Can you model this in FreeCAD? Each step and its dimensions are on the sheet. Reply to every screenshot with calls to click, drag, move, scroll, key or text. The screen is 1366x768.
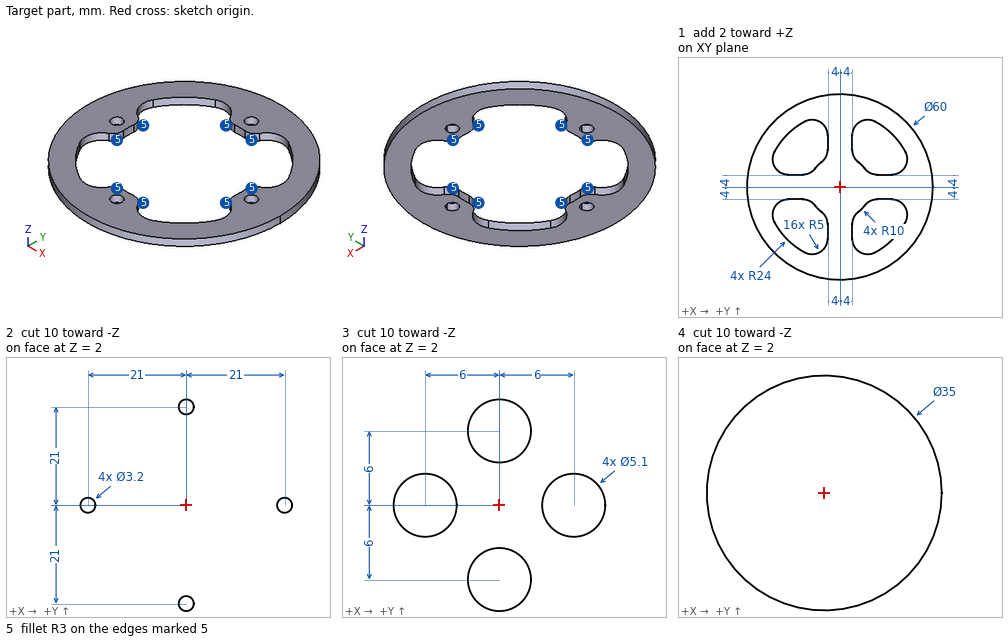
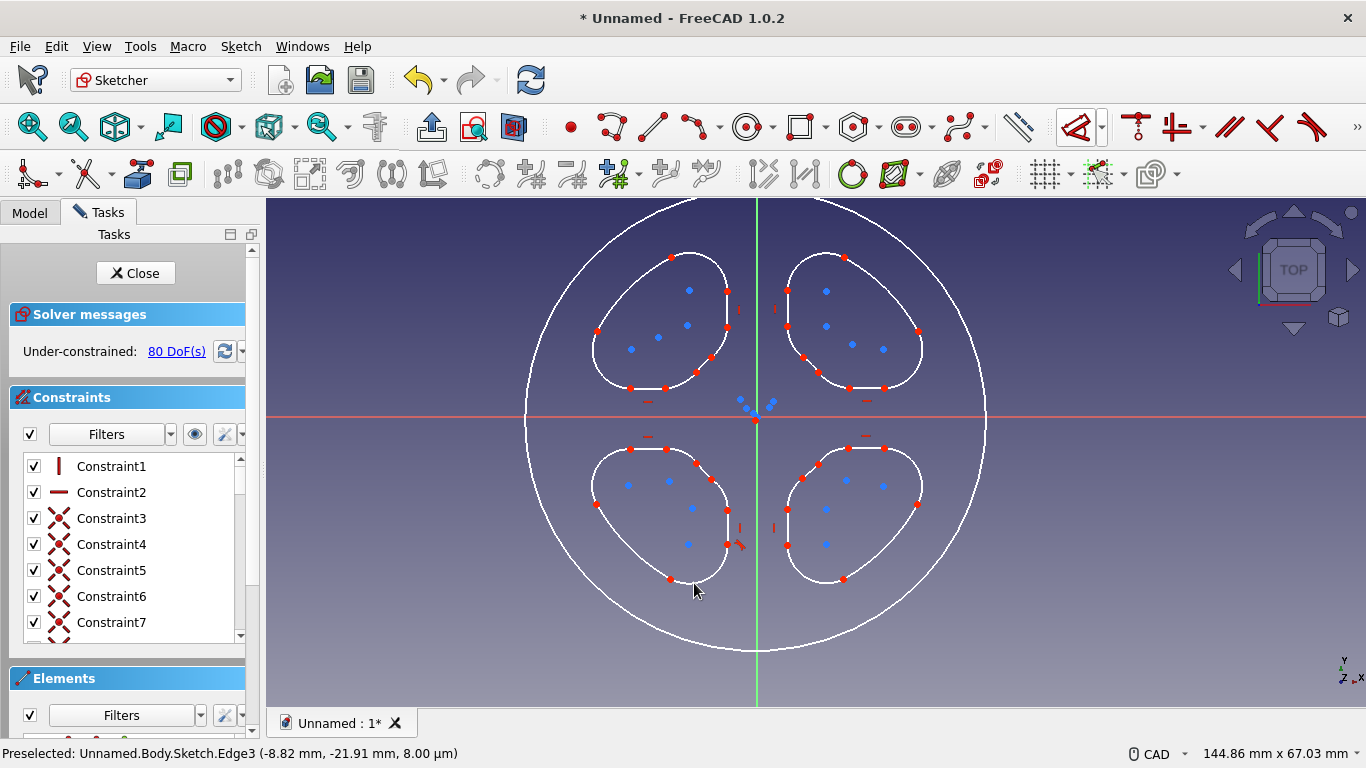
scroll(728, 521, up, 2)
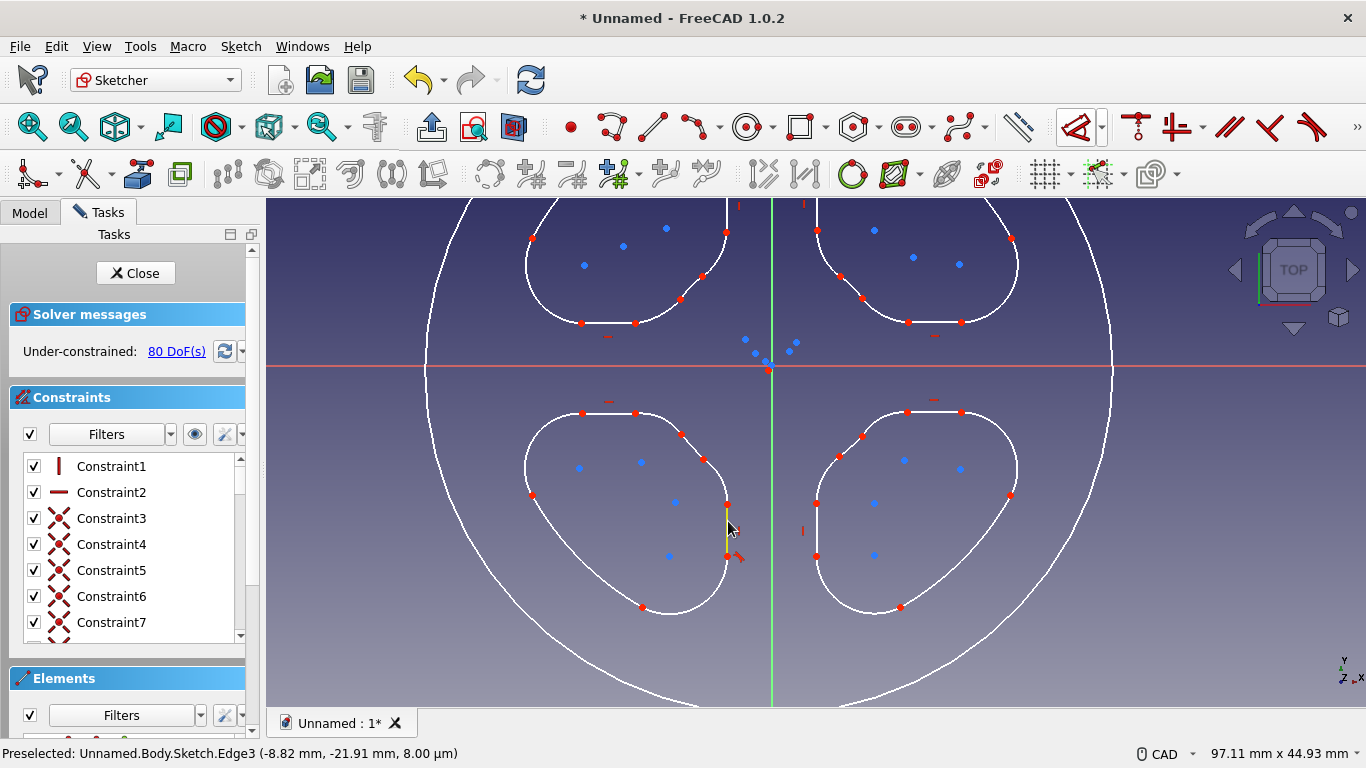
click(727, 520)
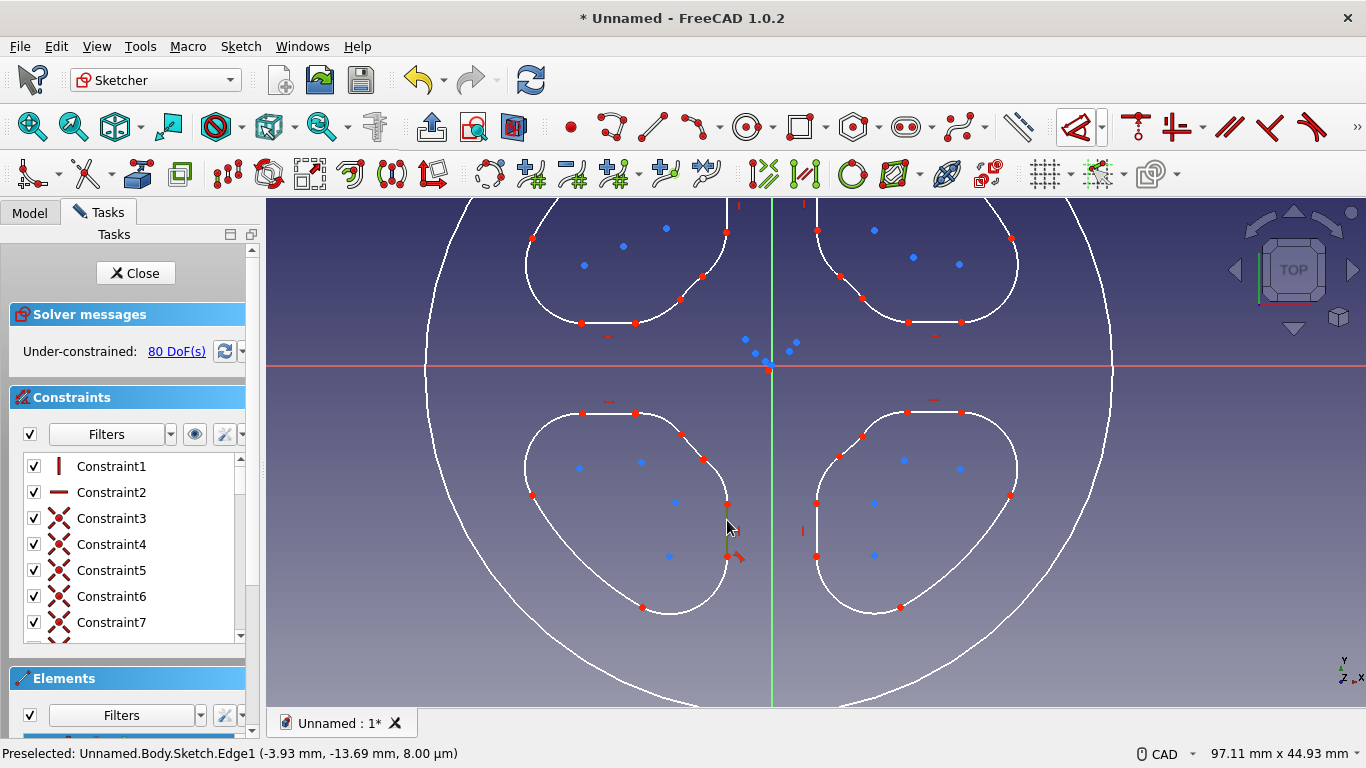
click(725, 489)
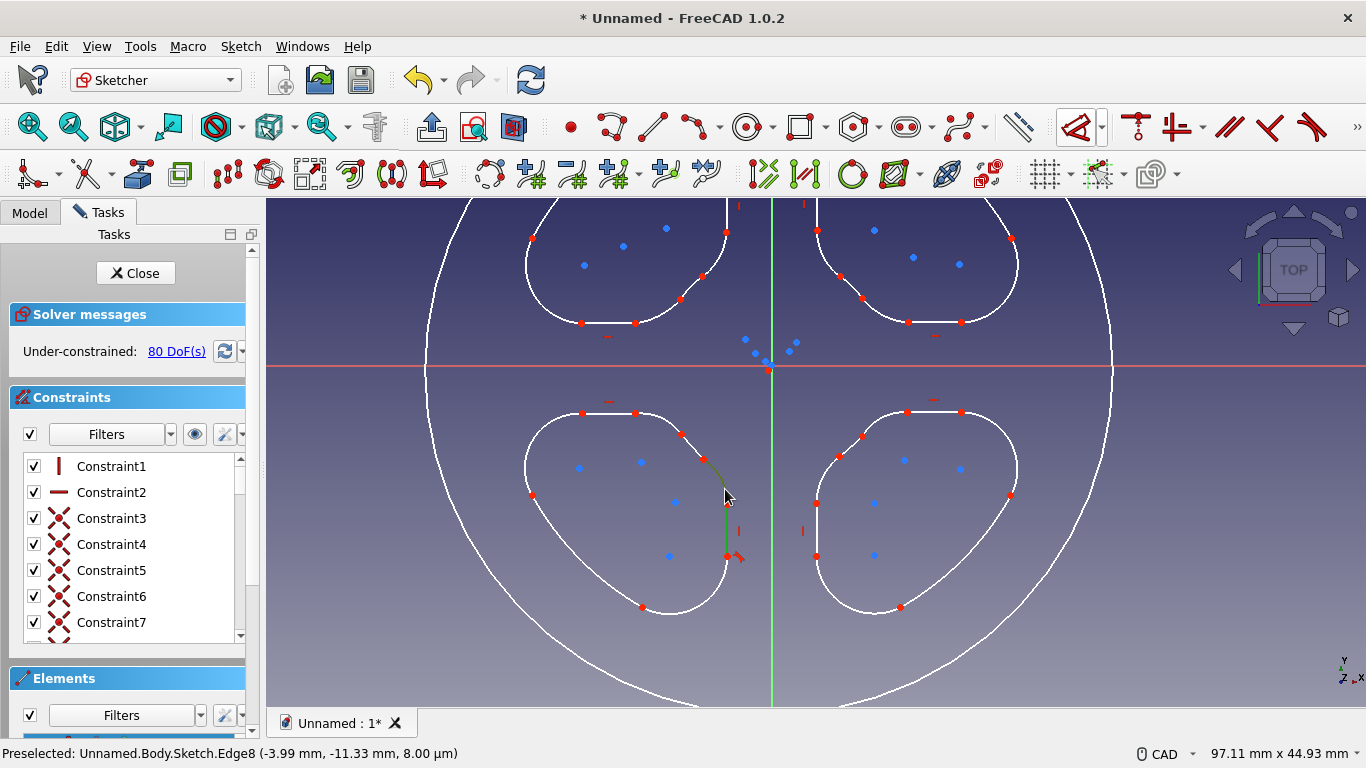
click(1312, 128)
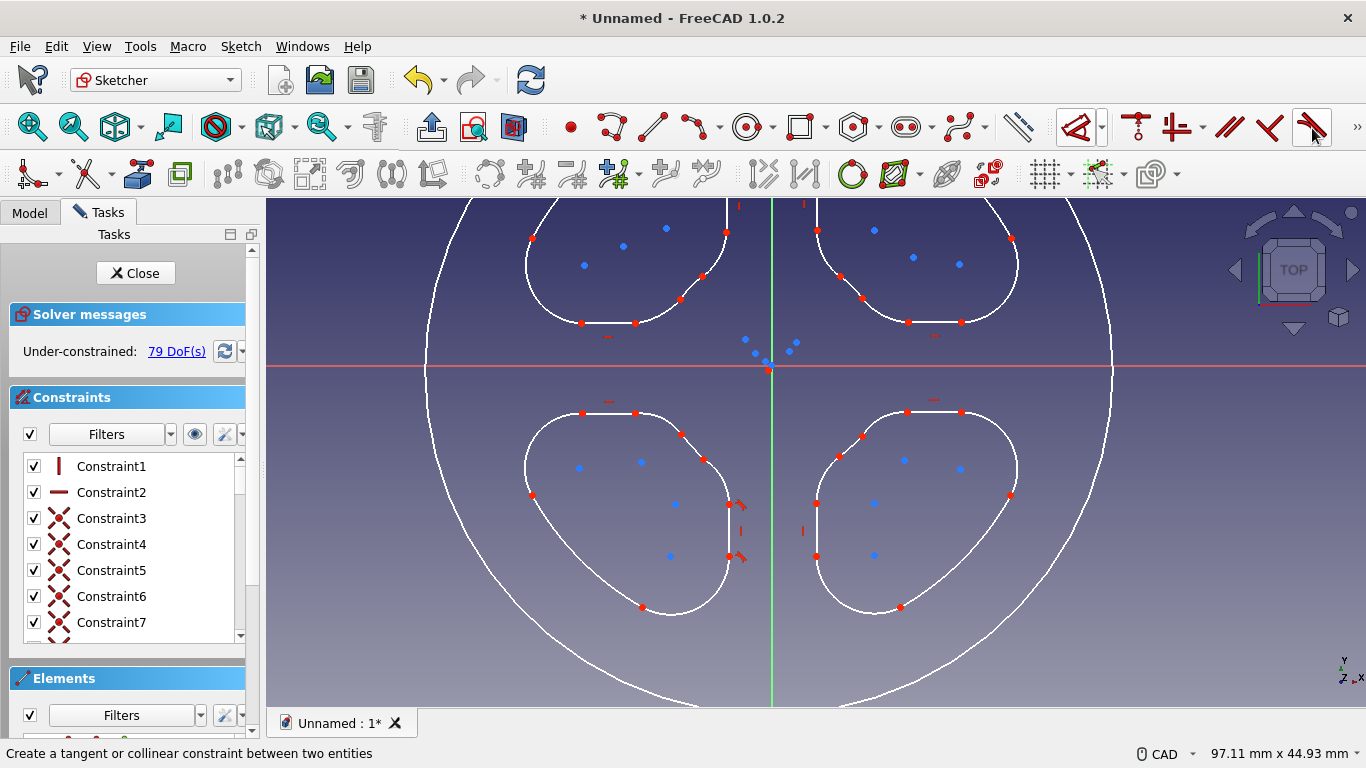
click(599, 414)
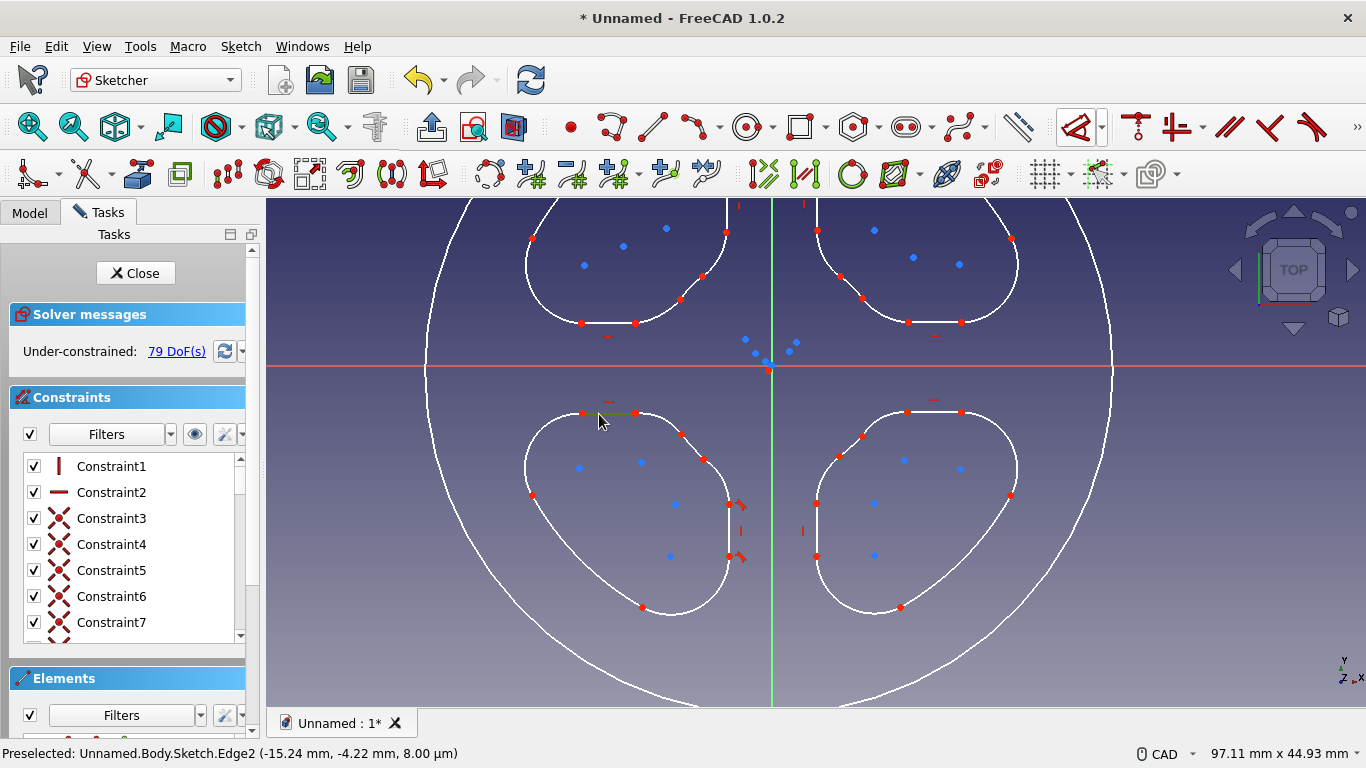
click(549, 423)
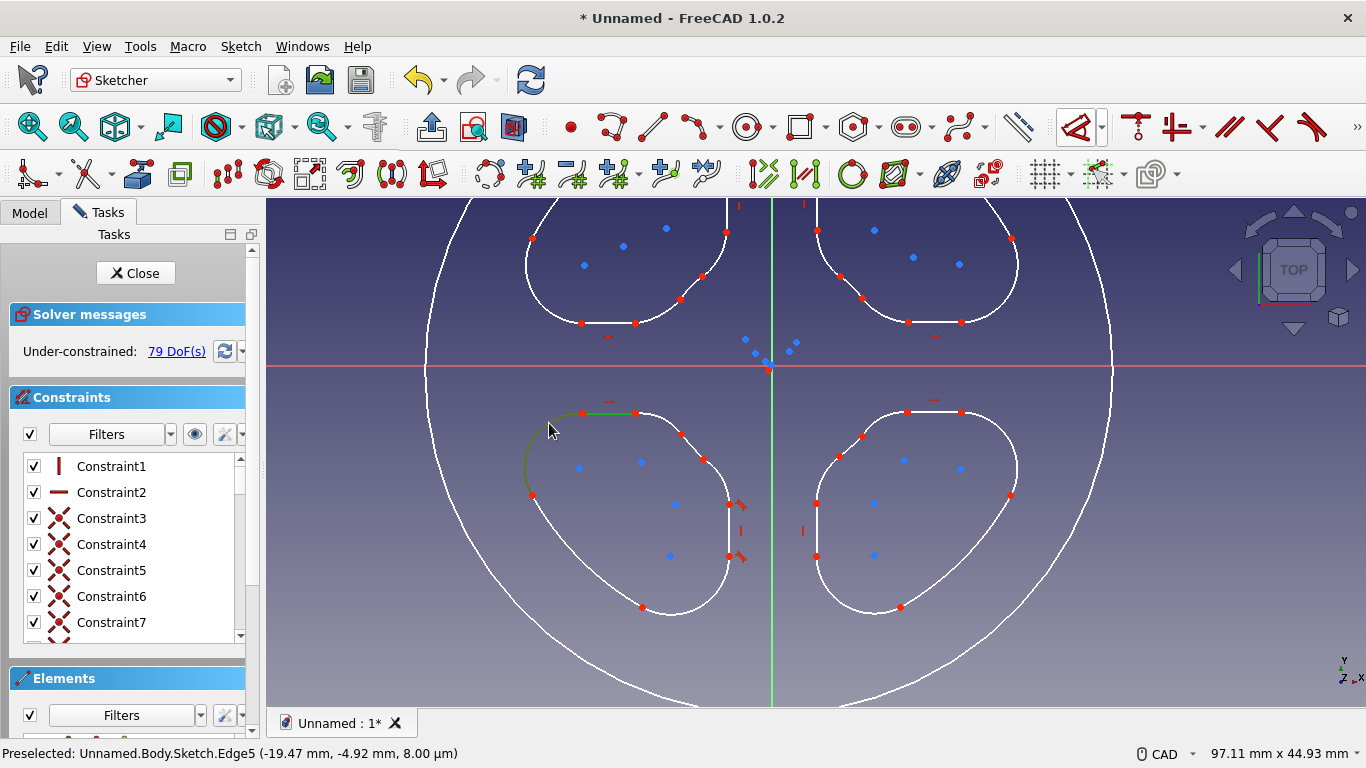
key(t)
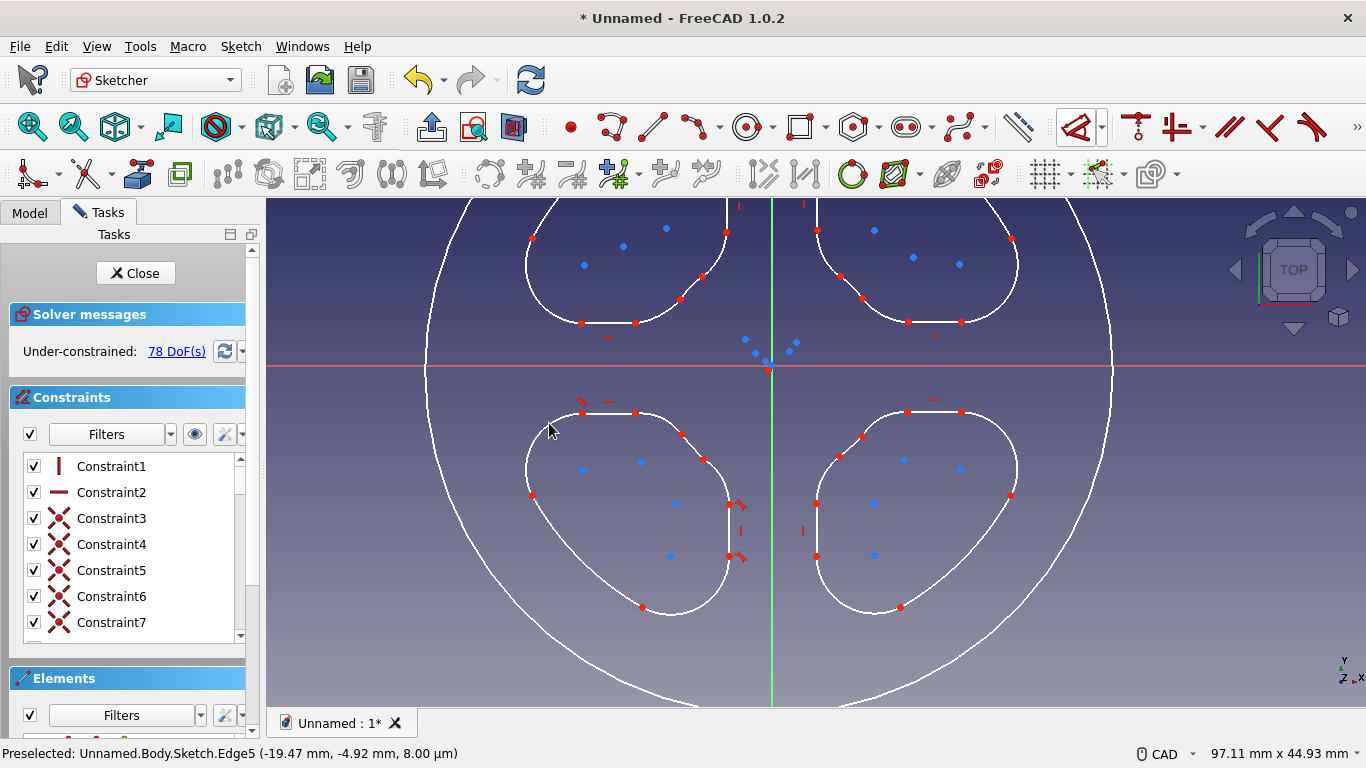
click(598, 414)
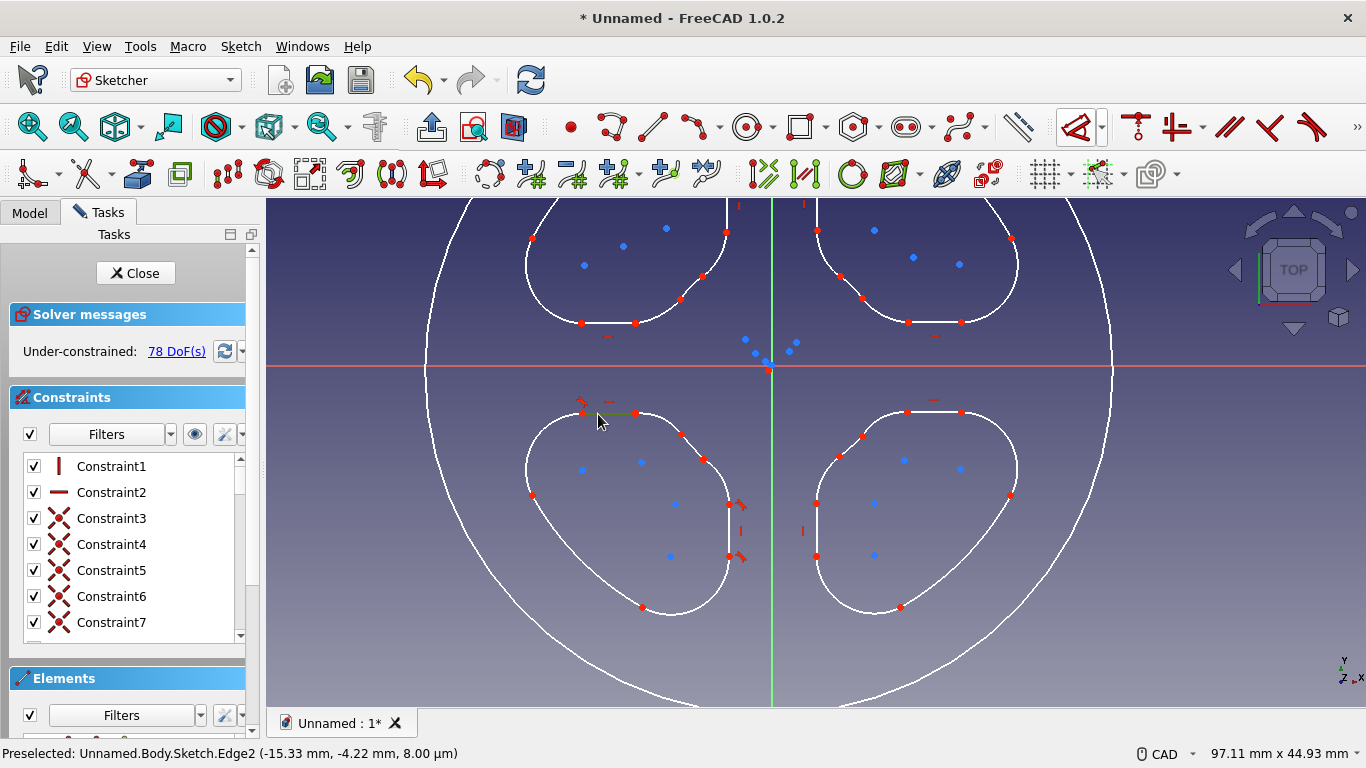
click(671, 423)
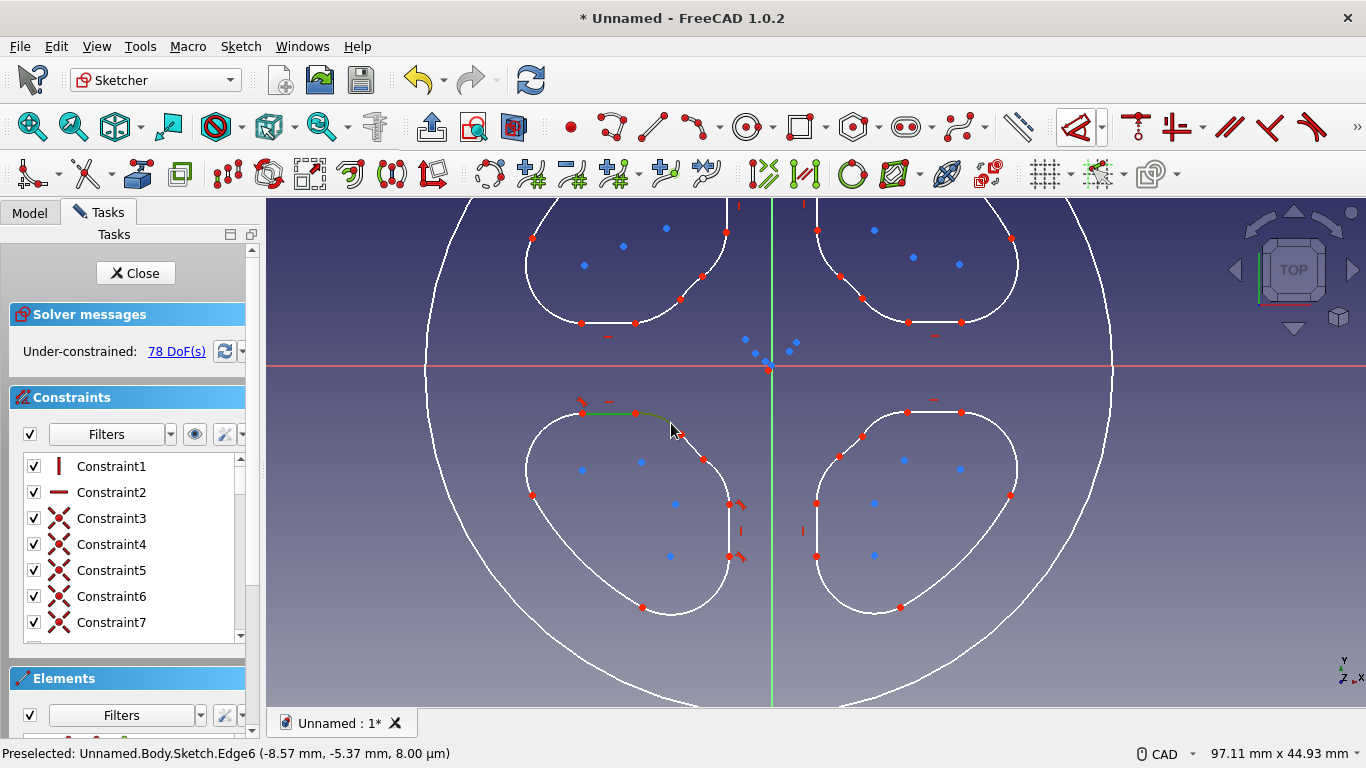
click(1312, 128)